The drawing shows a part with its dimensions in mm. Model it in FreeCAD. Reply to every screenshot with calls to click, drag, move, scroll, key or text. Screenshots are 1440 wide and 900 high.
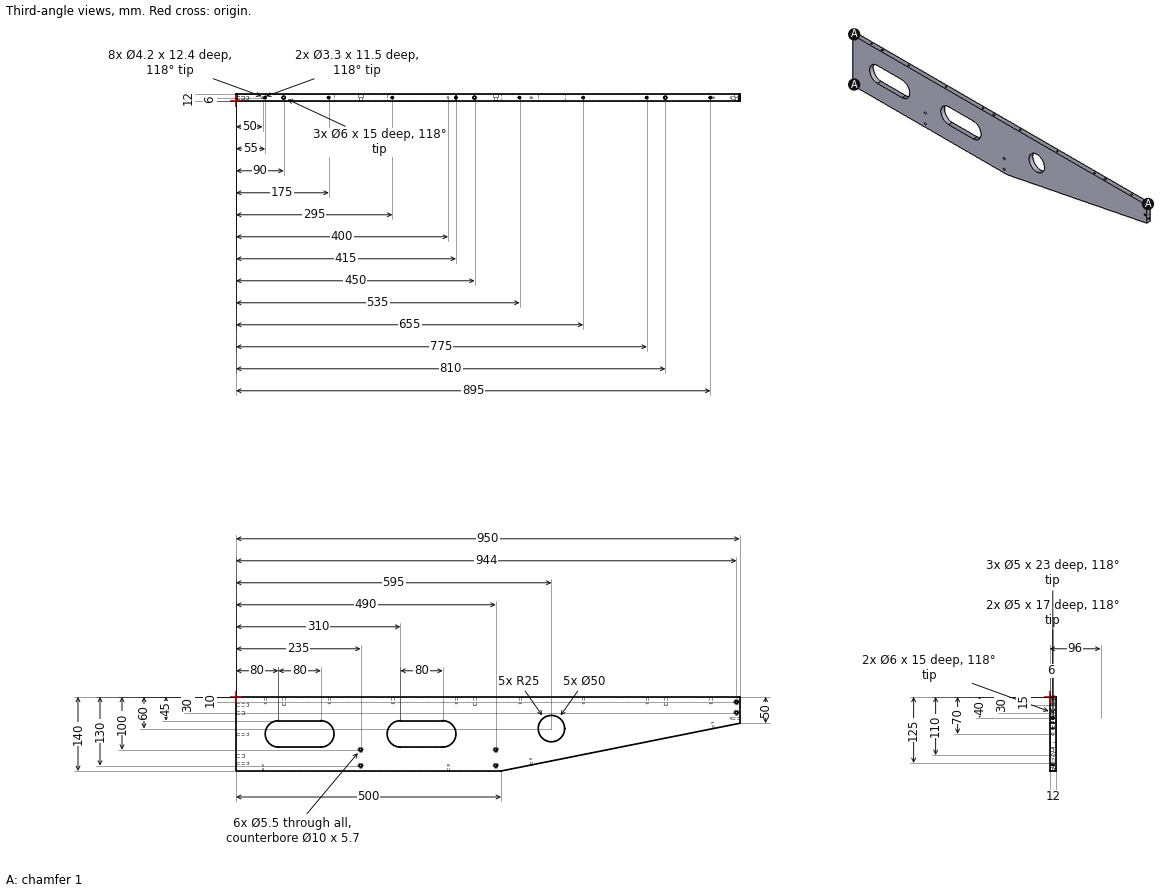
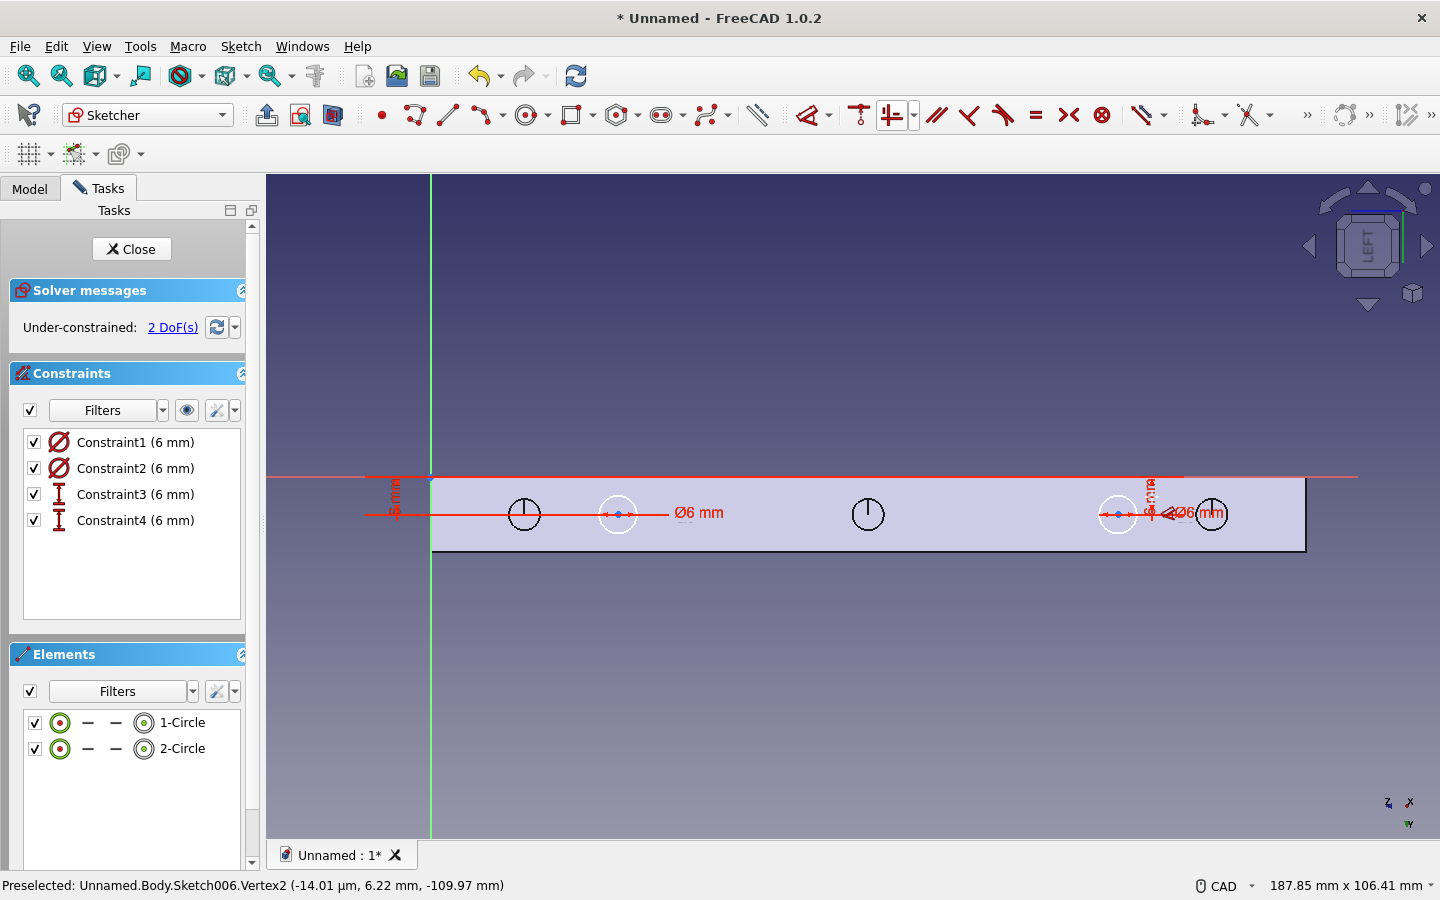
click(618, 515)
click(524, 443)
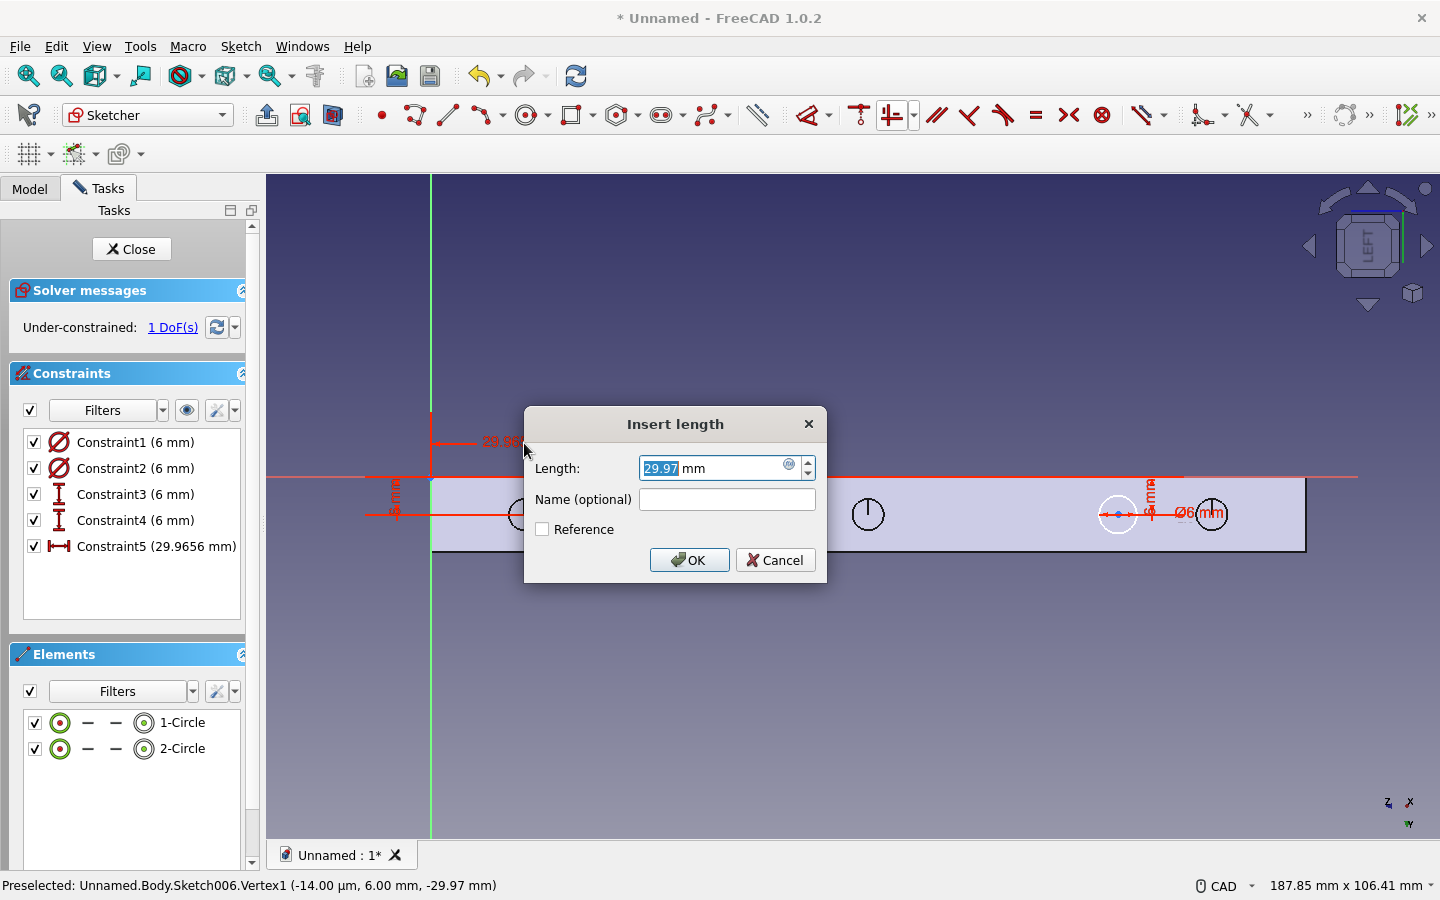
text(30)
key(Return)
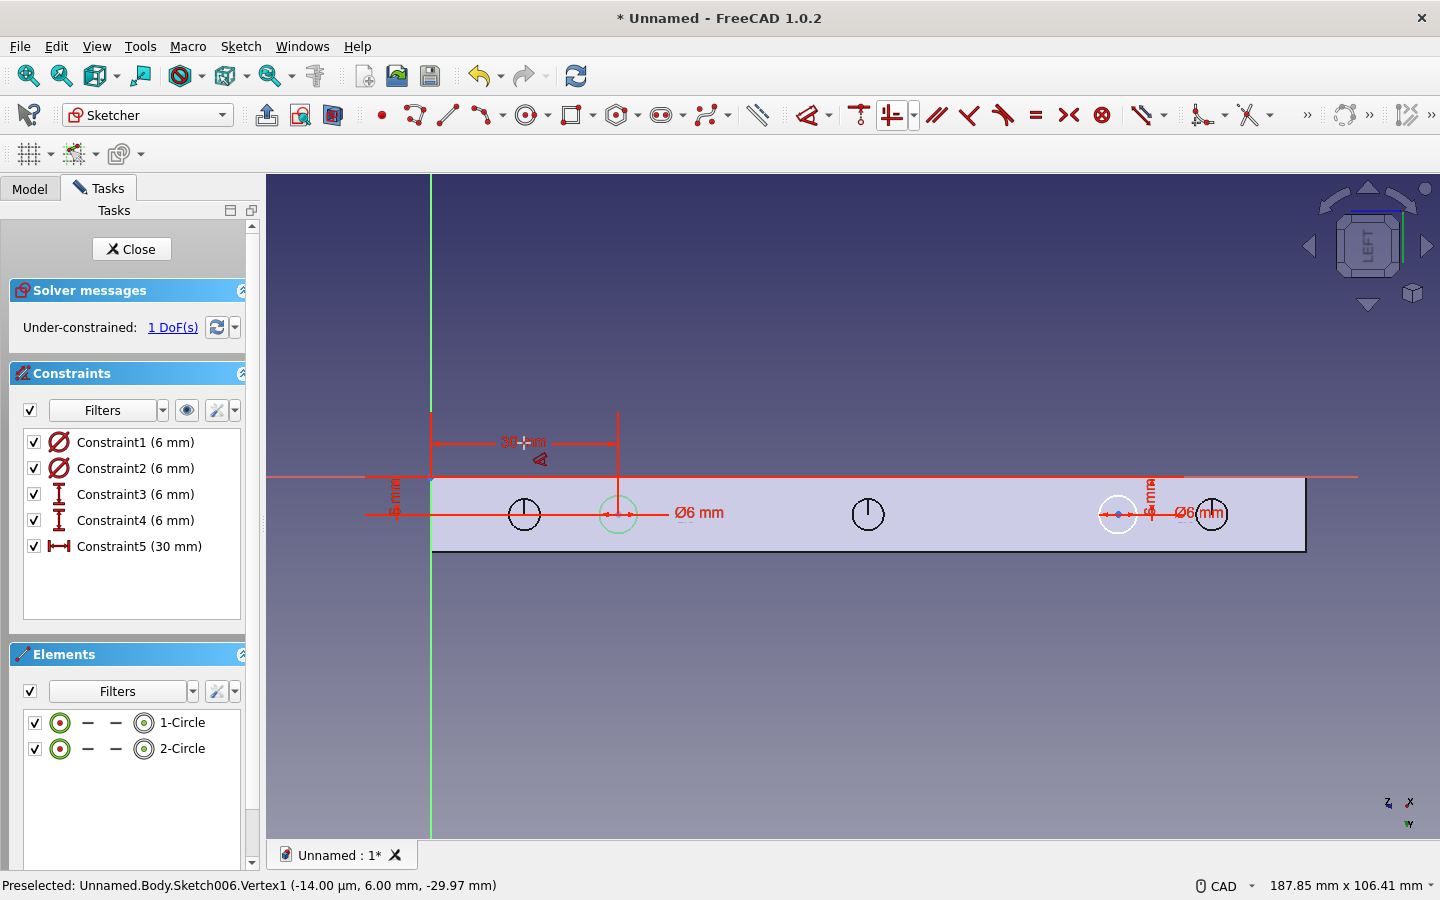
click(1118, 515)
click(774, 443)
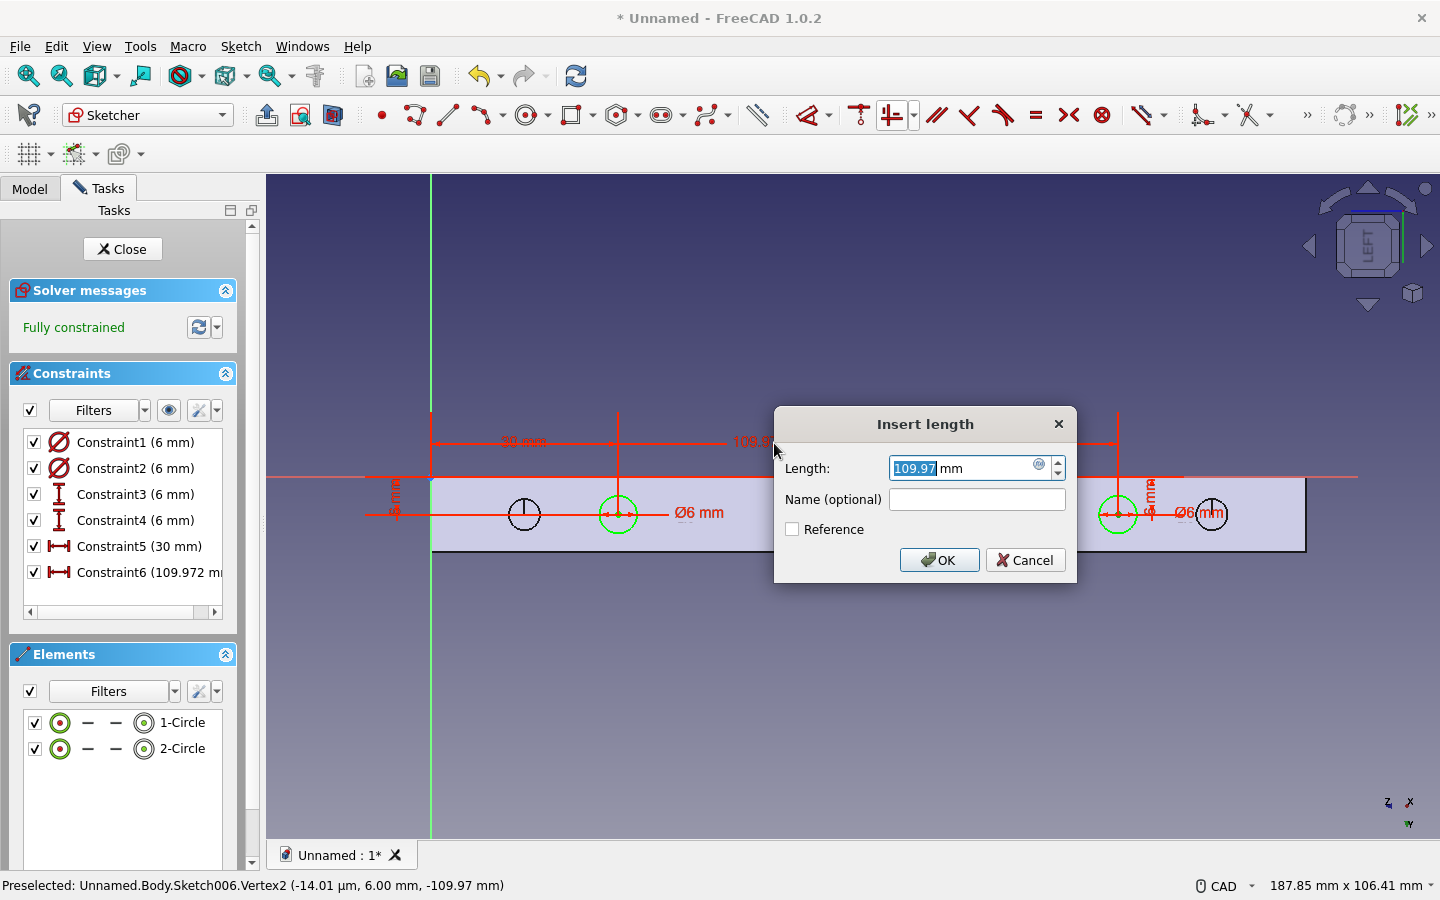
text(110)
key(Return)
key(Escape)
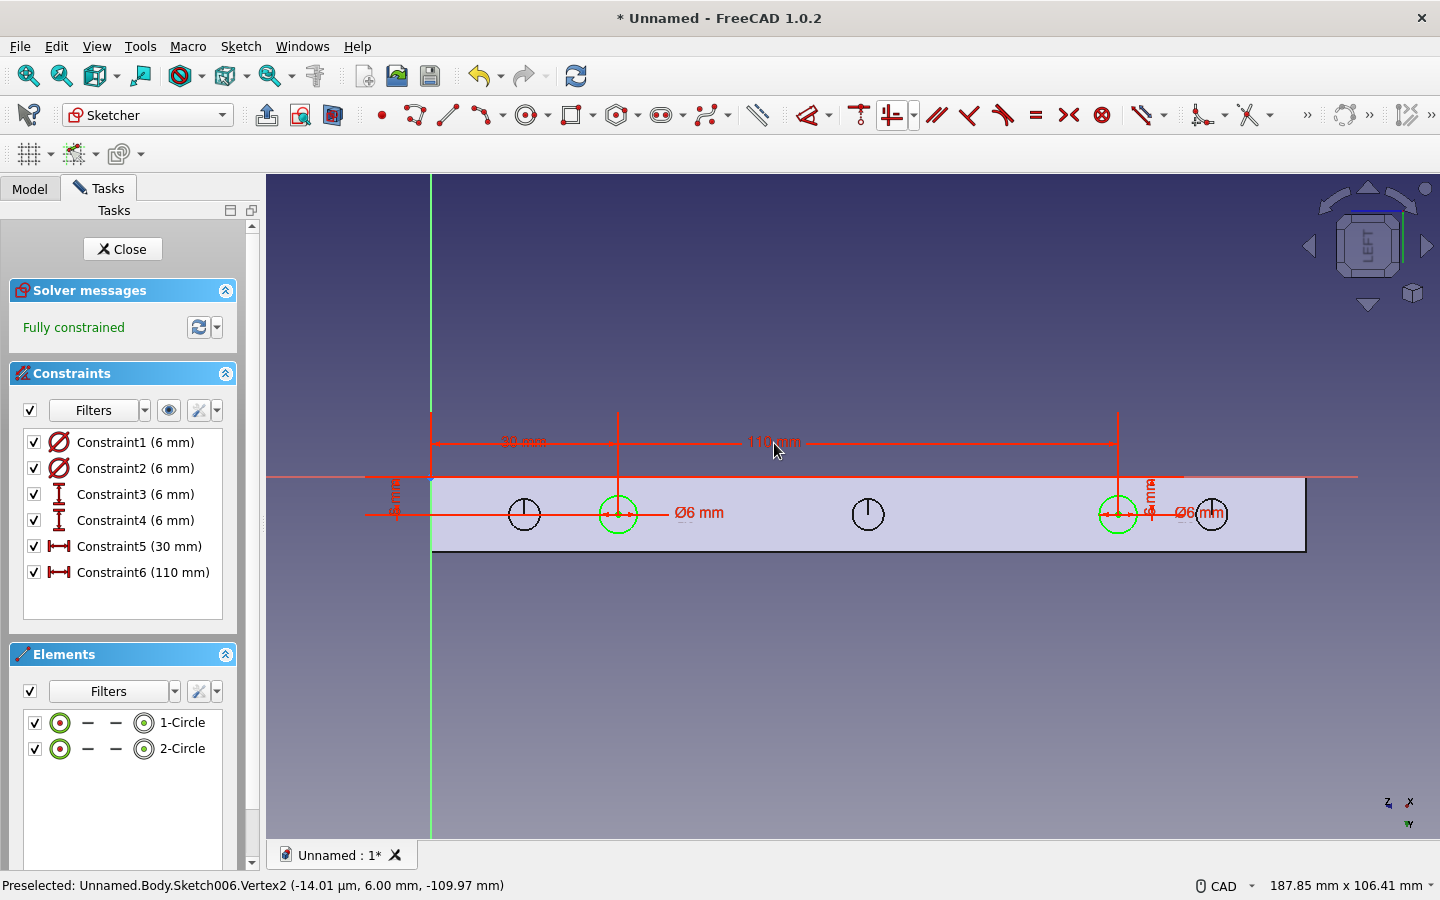
click(123, 249)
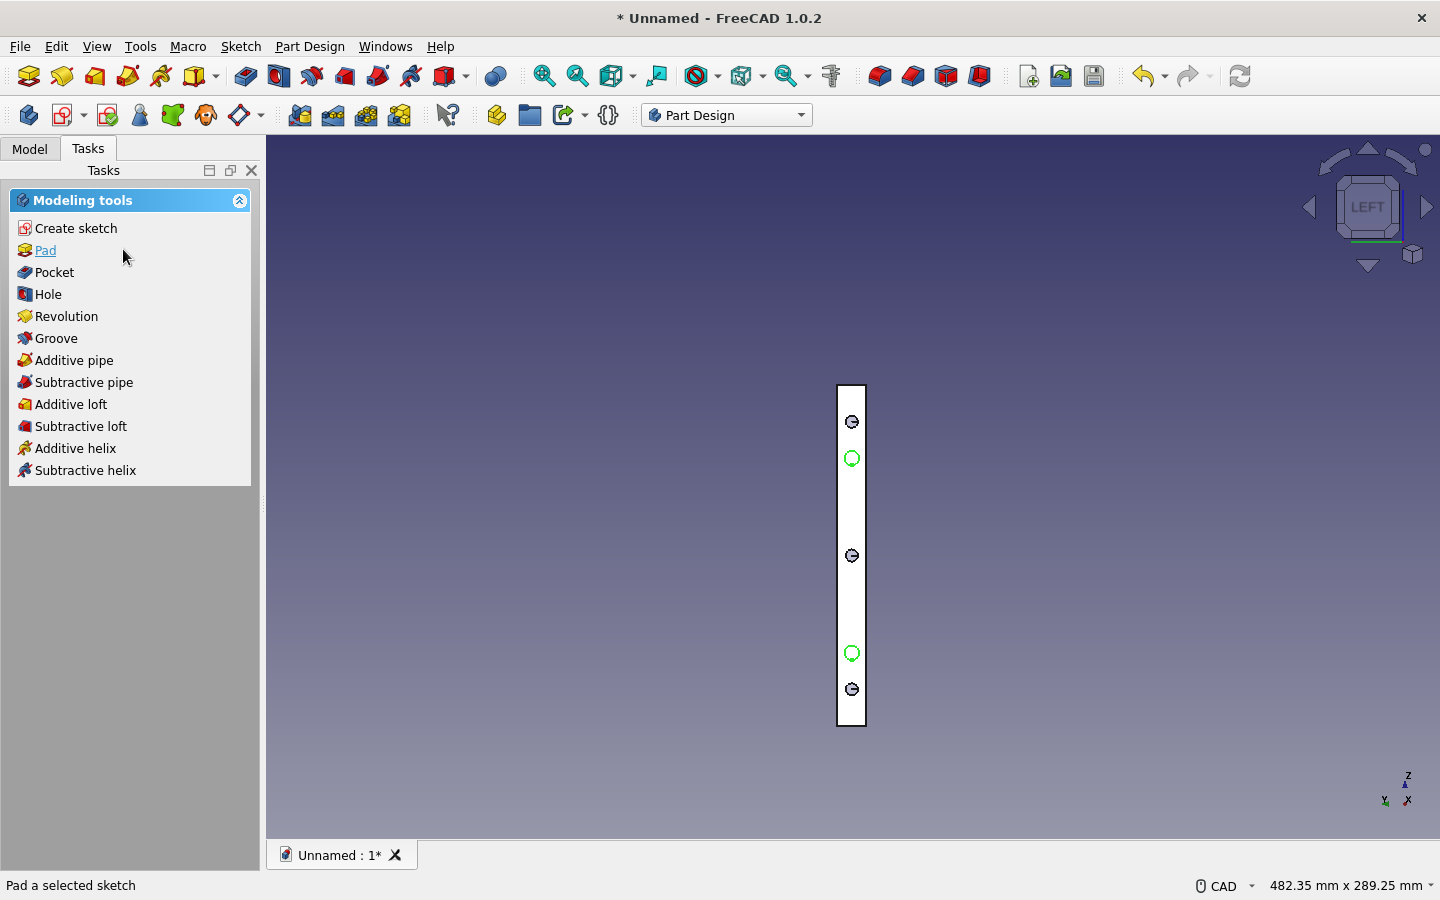
click(279, 76)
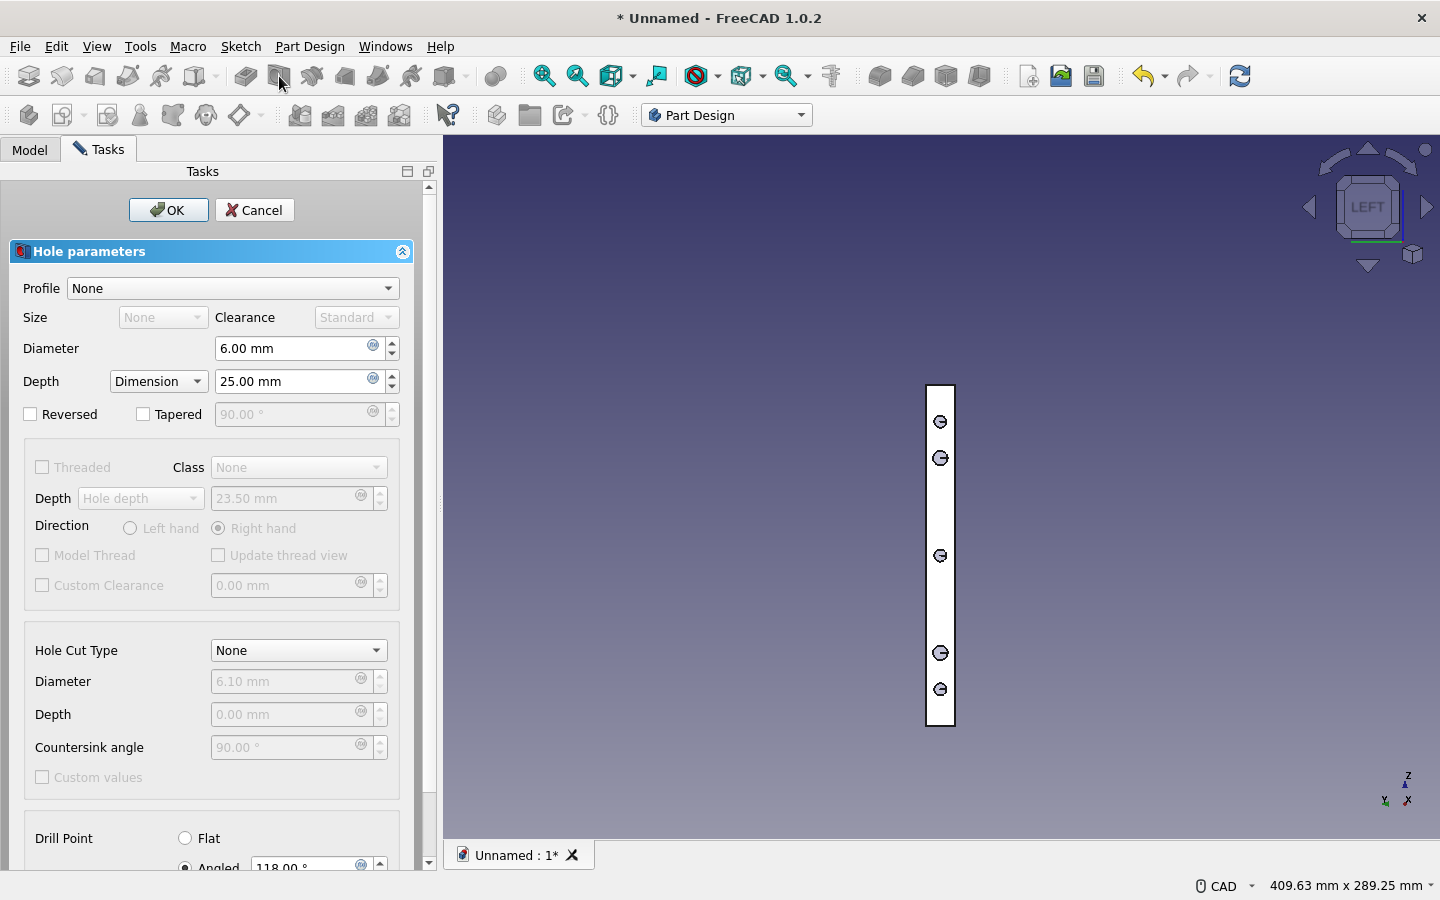
triple_click(300, 348)